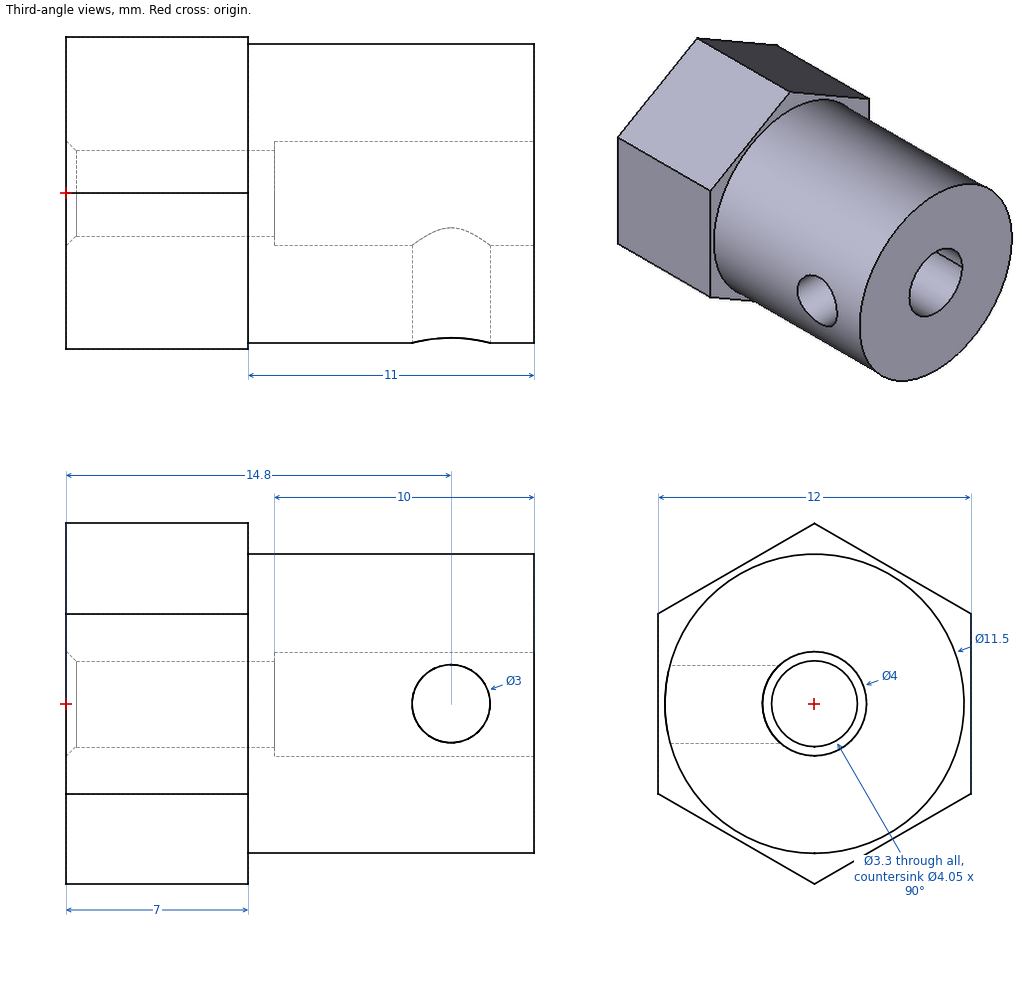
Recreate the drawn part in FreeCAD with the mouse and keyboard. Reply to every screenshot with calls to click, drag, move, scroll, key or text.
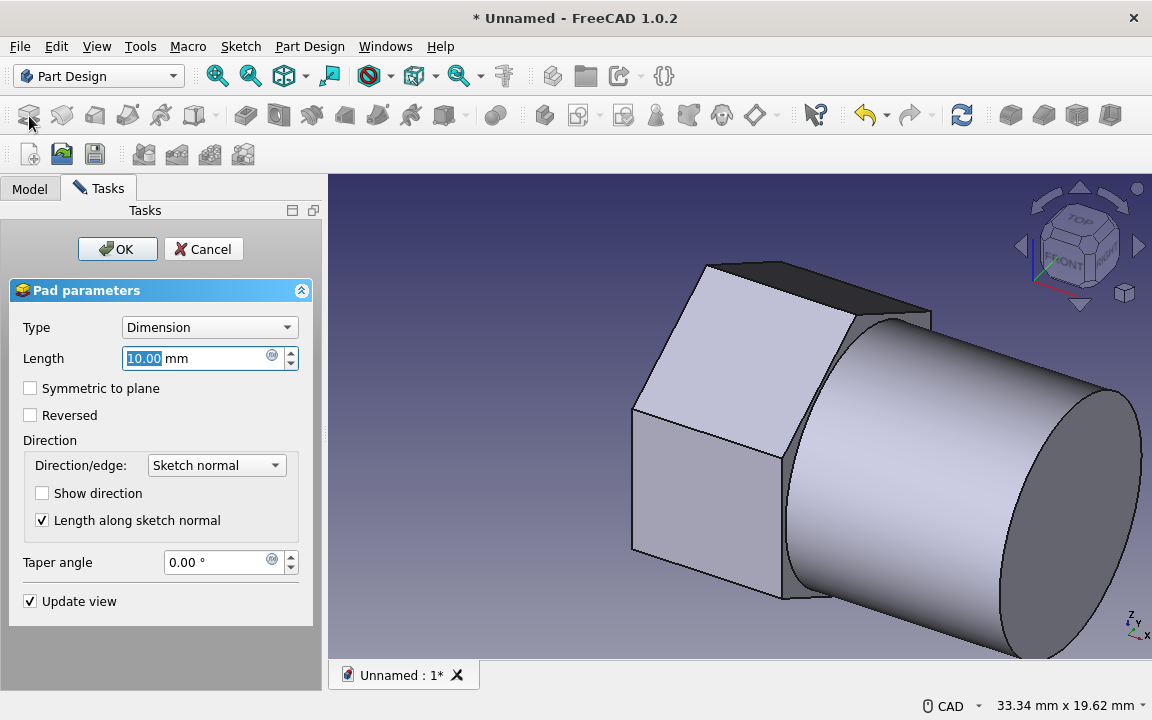
text(11)
key(Tab)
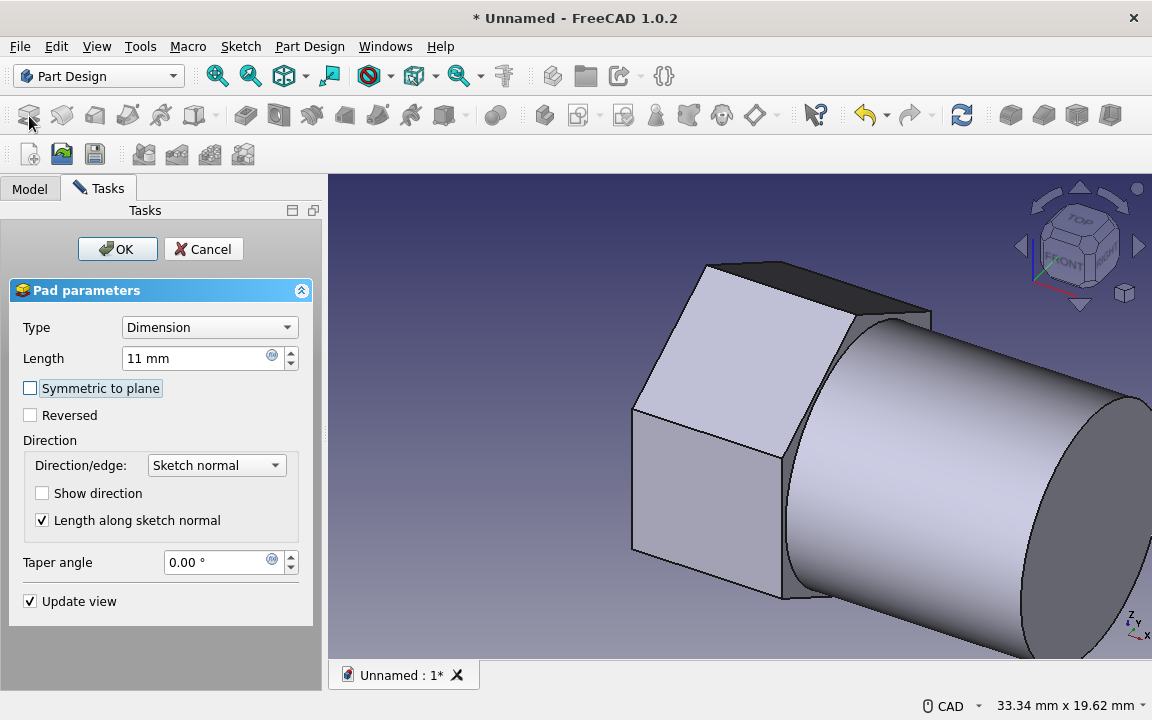
click(118, 249)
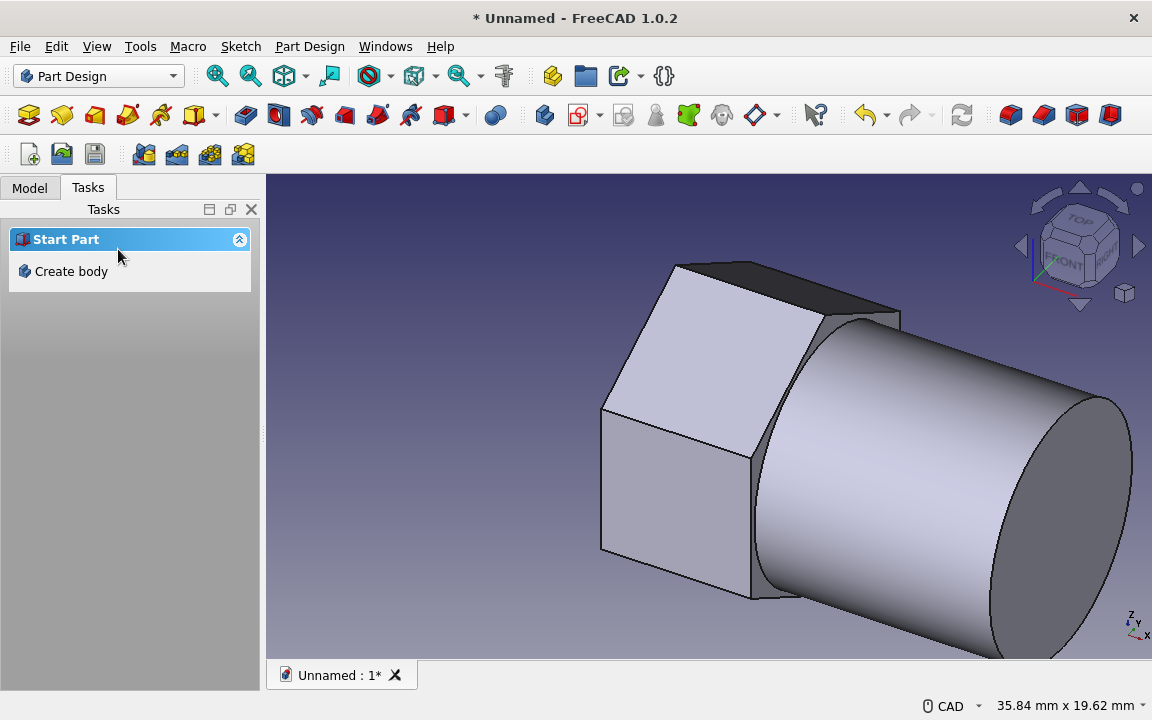
click(218, 76)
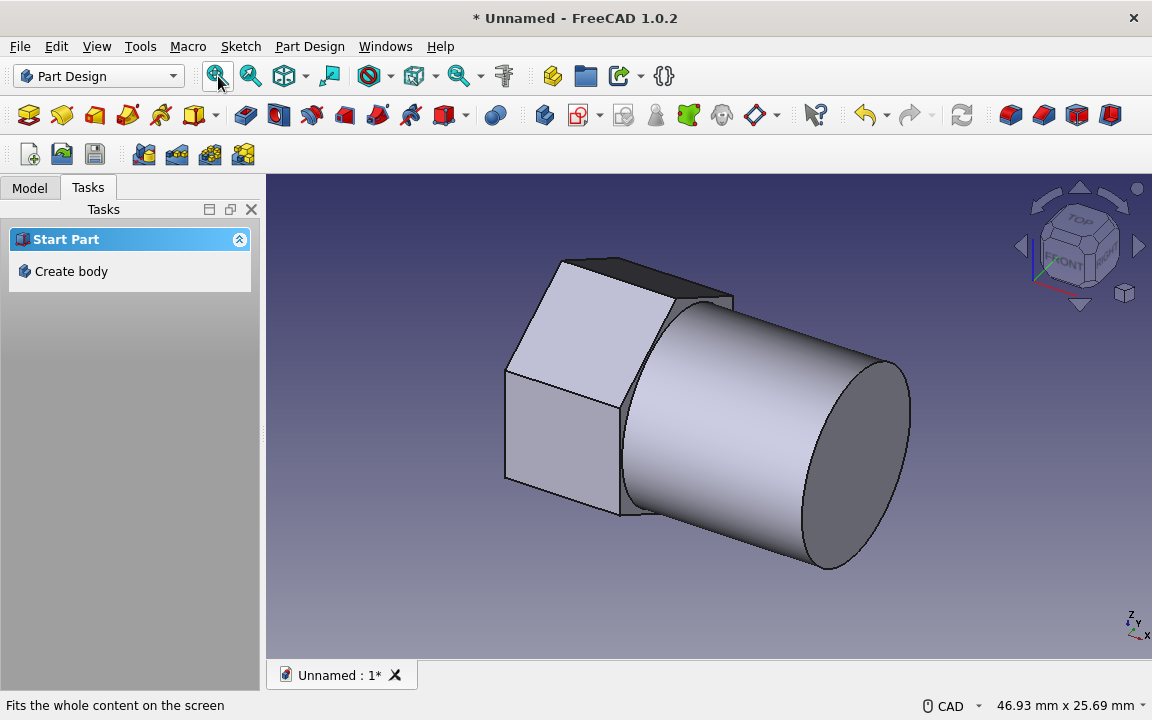
click(856, 464)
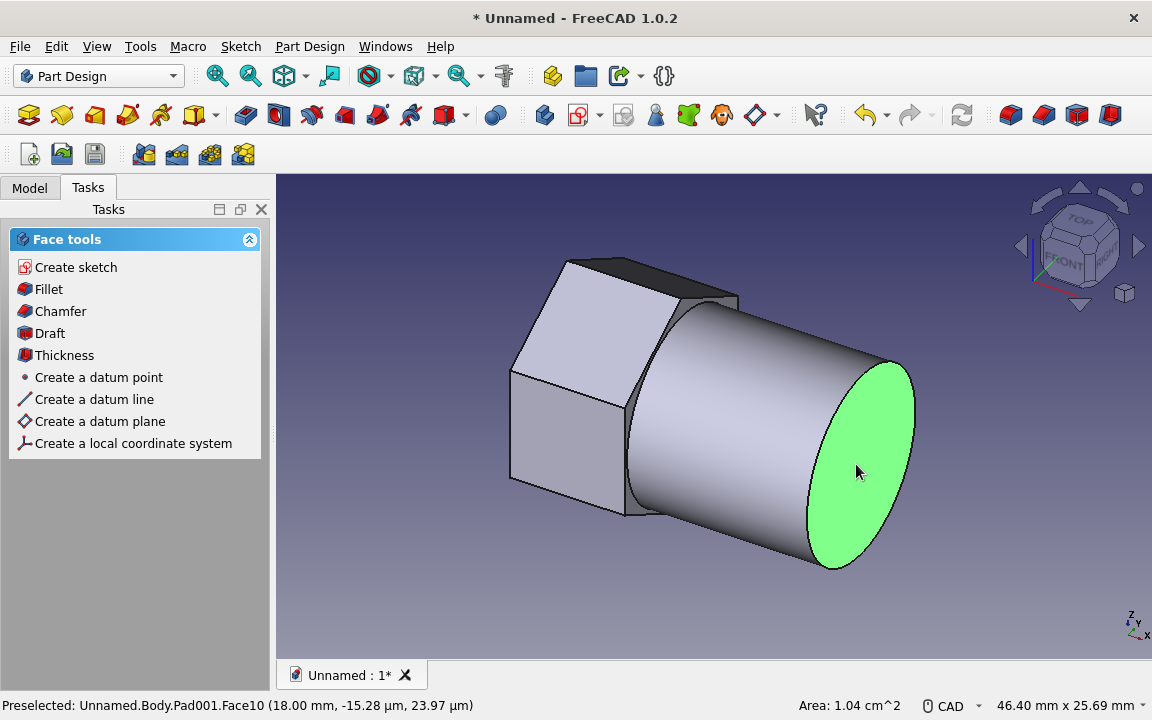
click(578, 116)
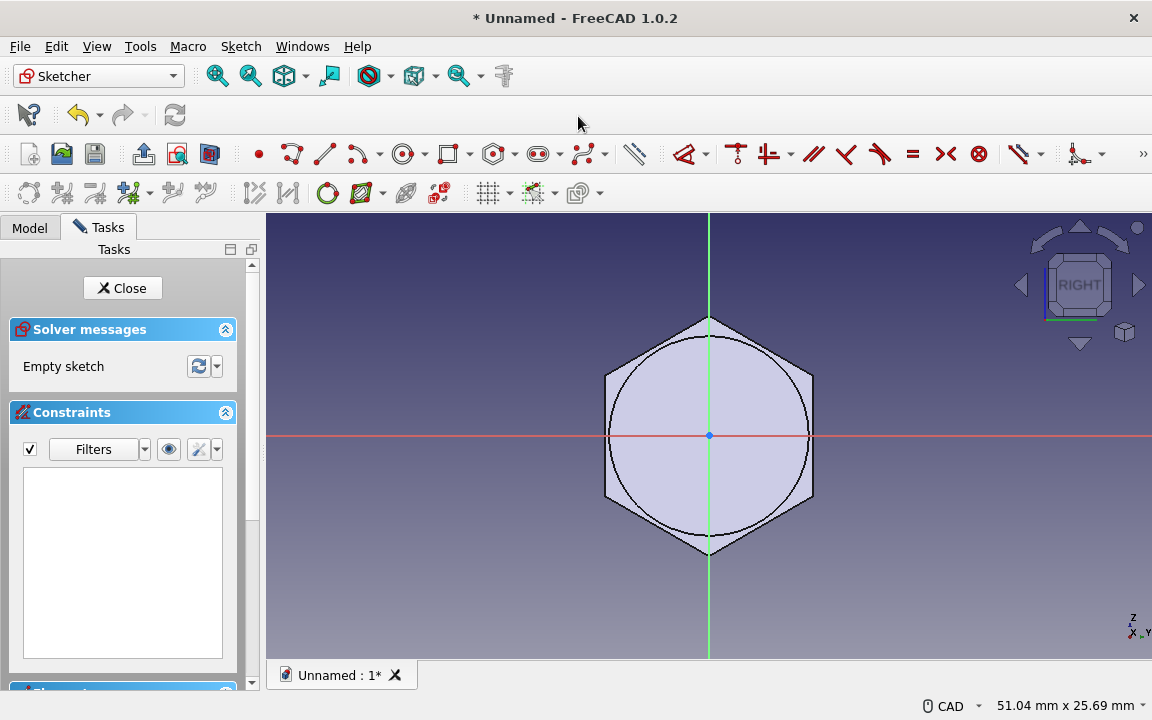
scroll(731, 436, up, 7)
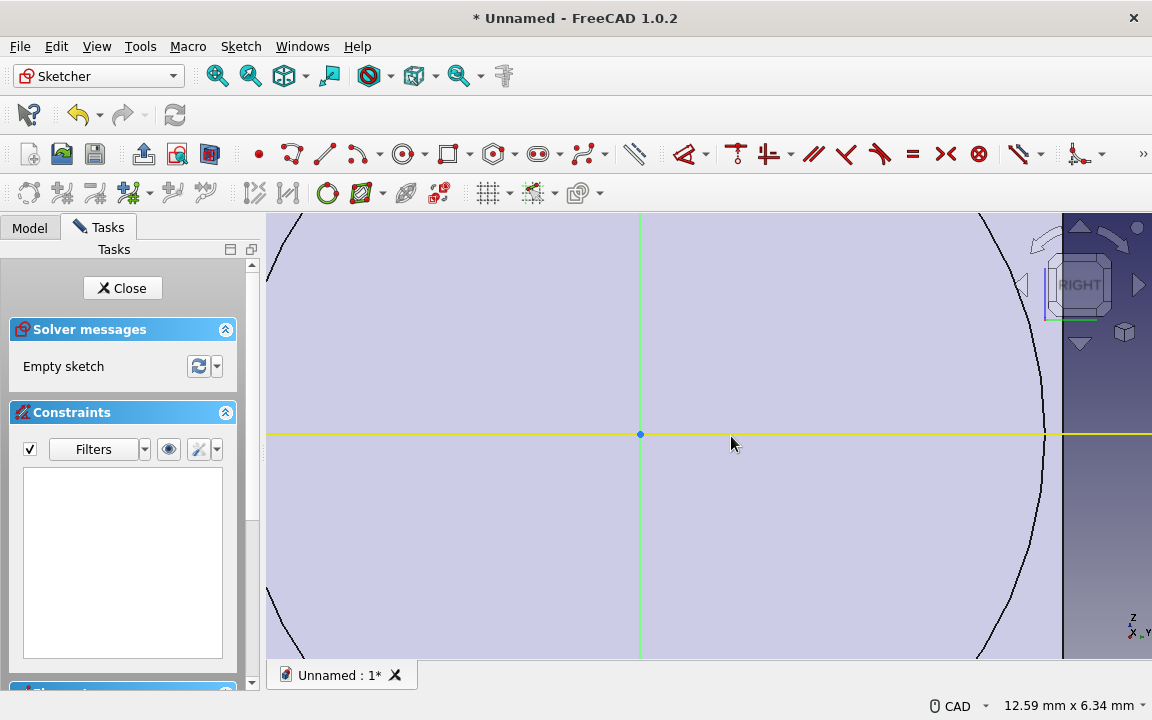
click(402, 154)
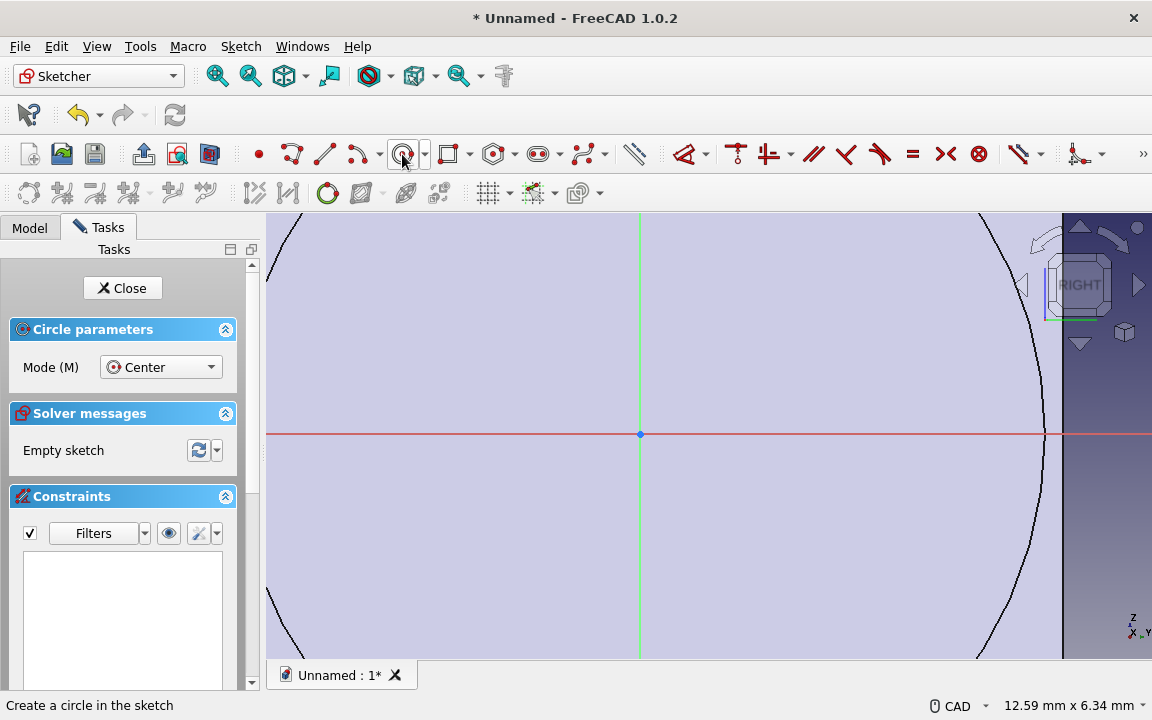
click(640, 434)
move(740, 335)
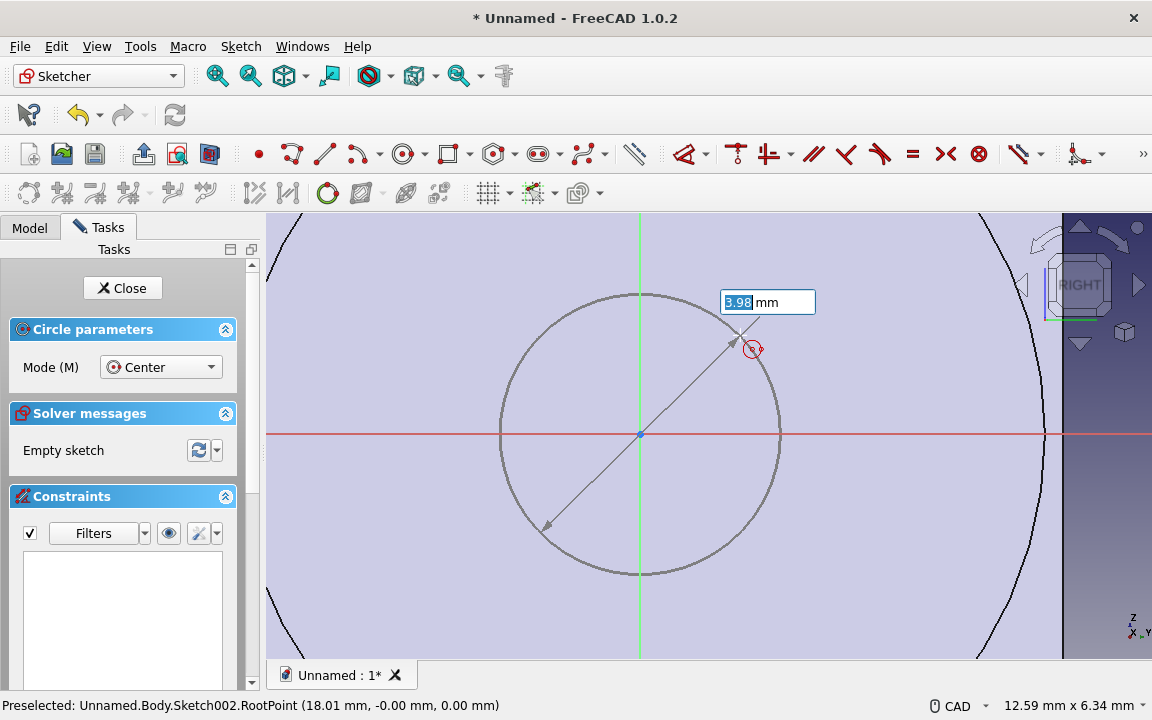
text(4)
key(Return)
key(Escape)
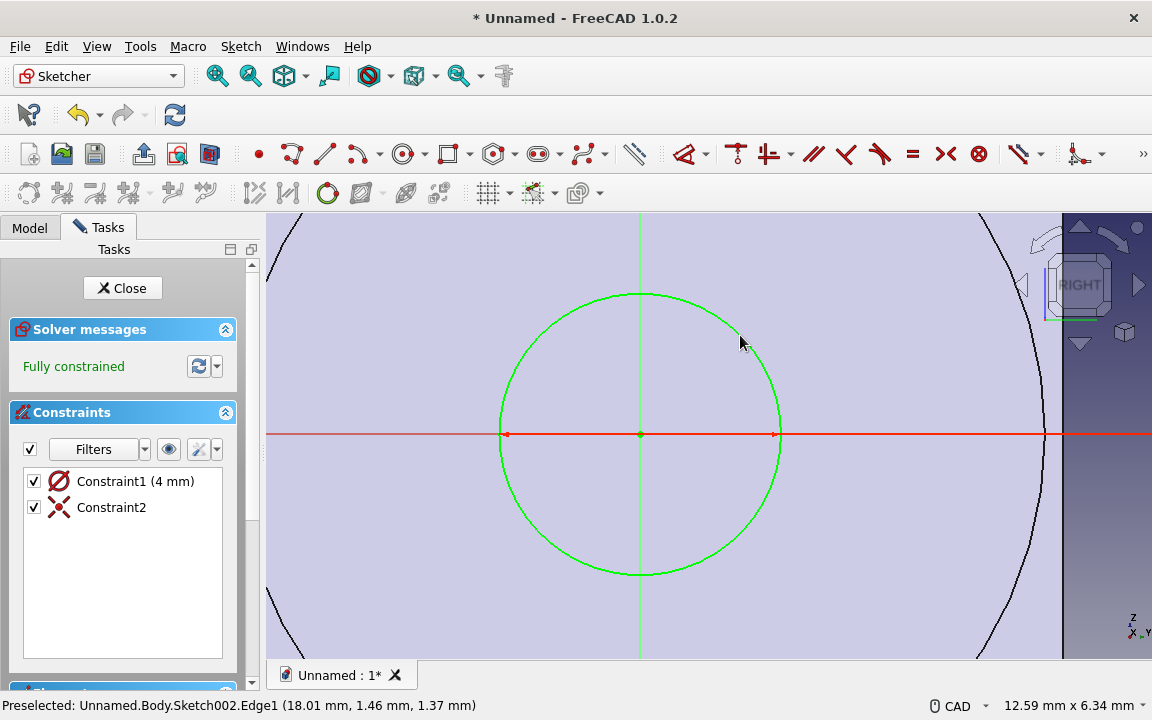
click(123, 288)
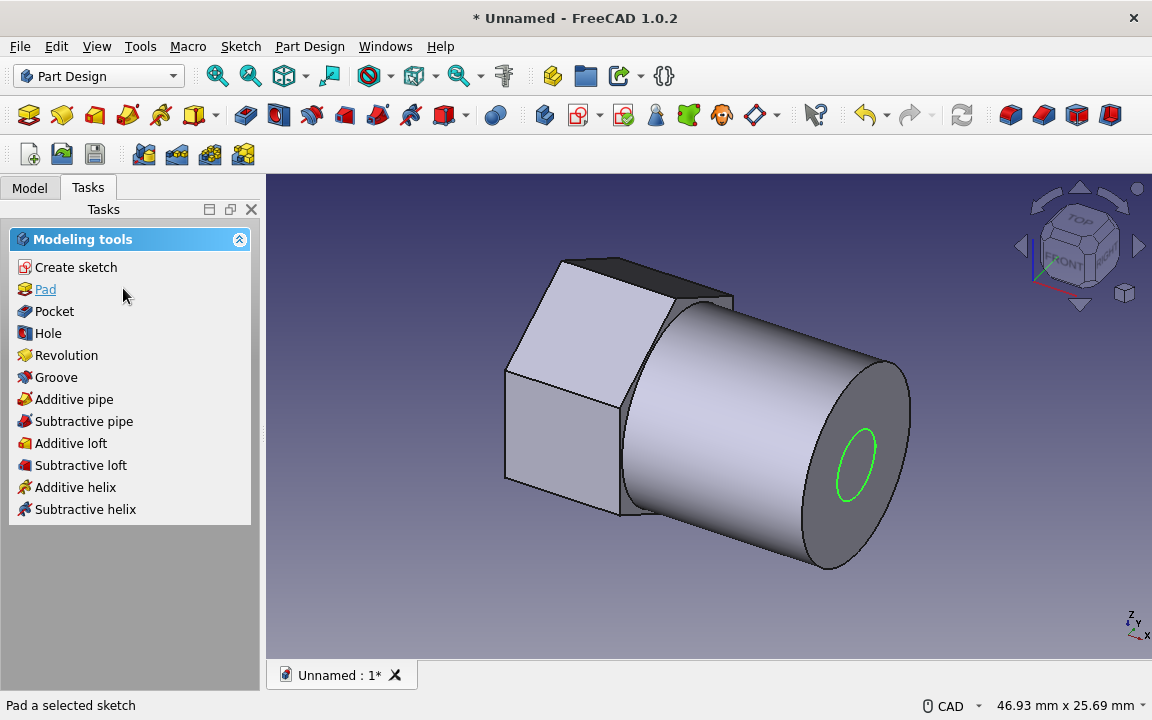
click(246, 116)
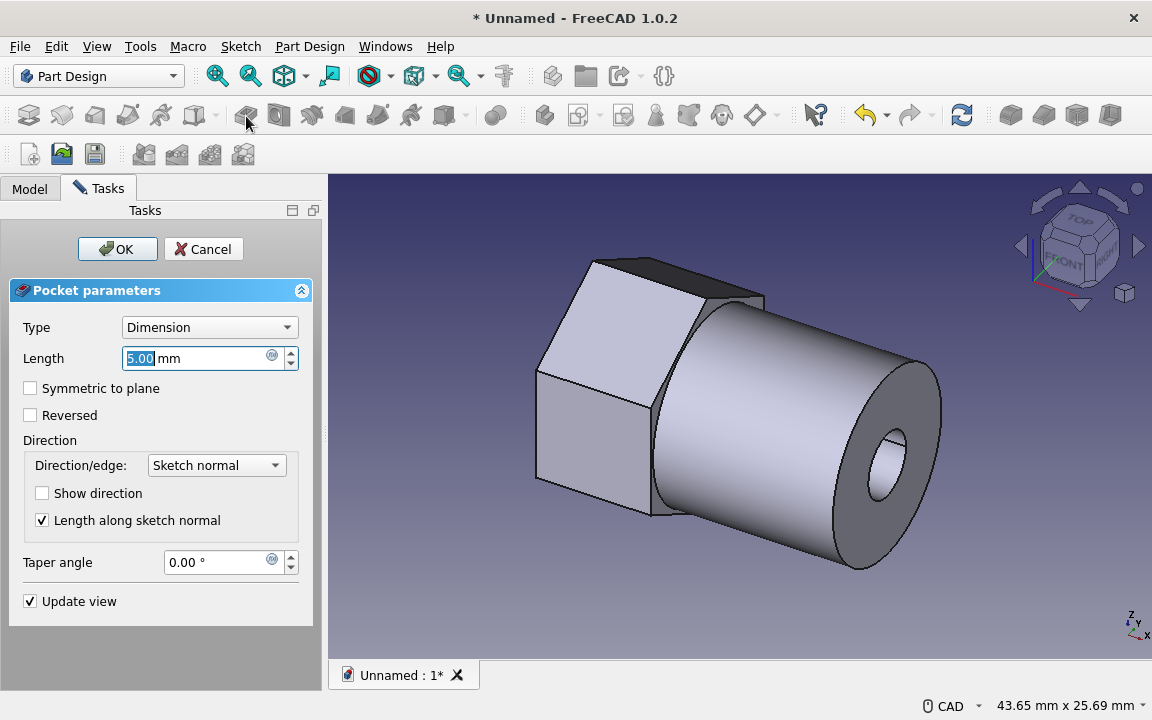
text(10)
key(Tab)